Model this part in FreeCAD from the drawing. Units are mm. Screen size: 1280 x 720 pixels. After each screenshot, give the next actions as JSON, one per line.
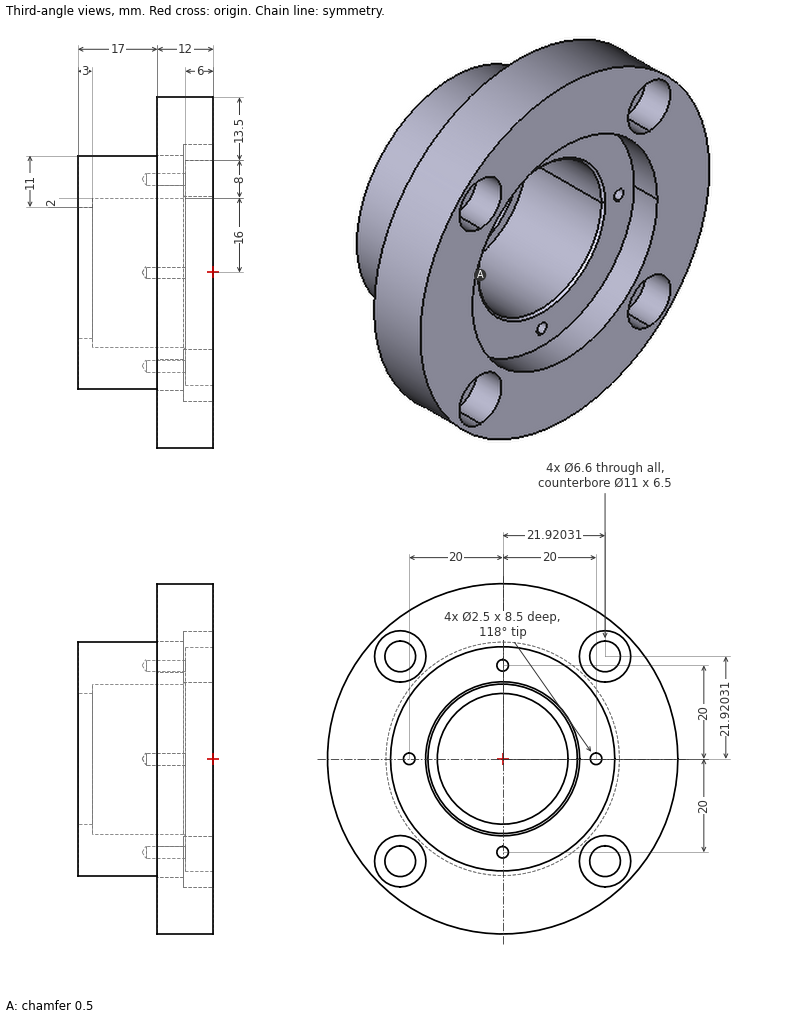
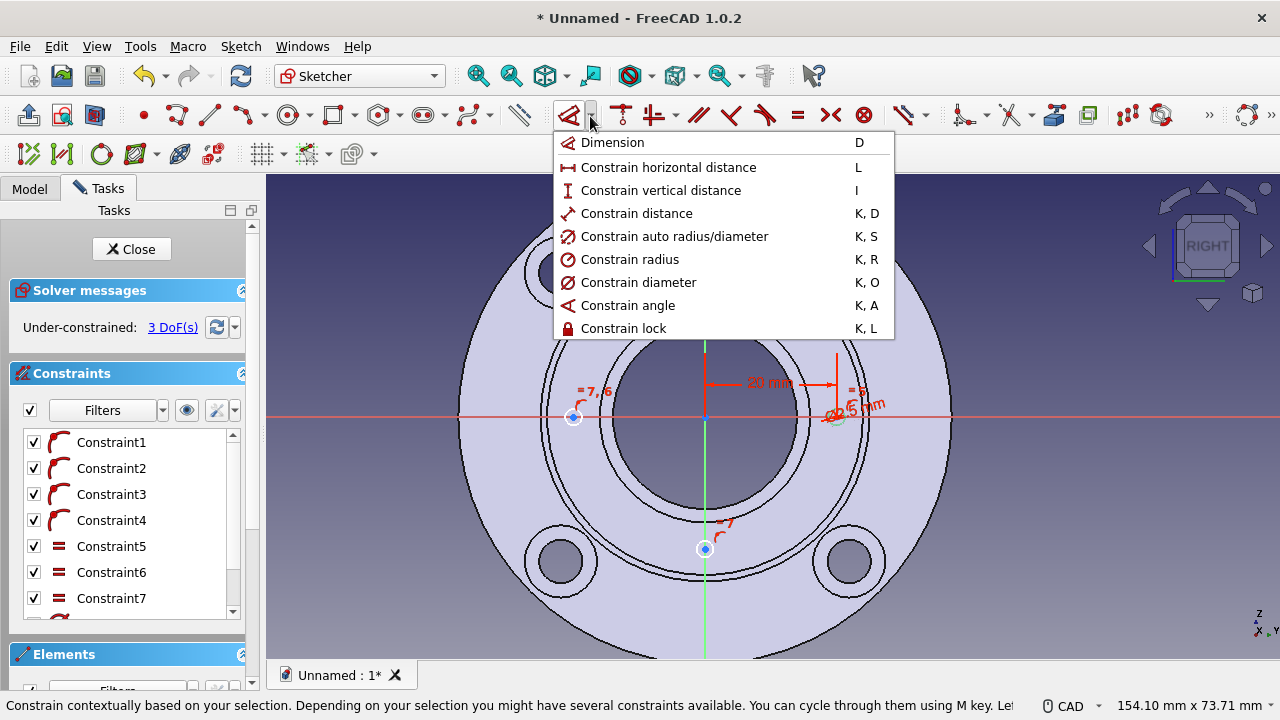
{"action": "left_click", "coordinate": [724, 190]}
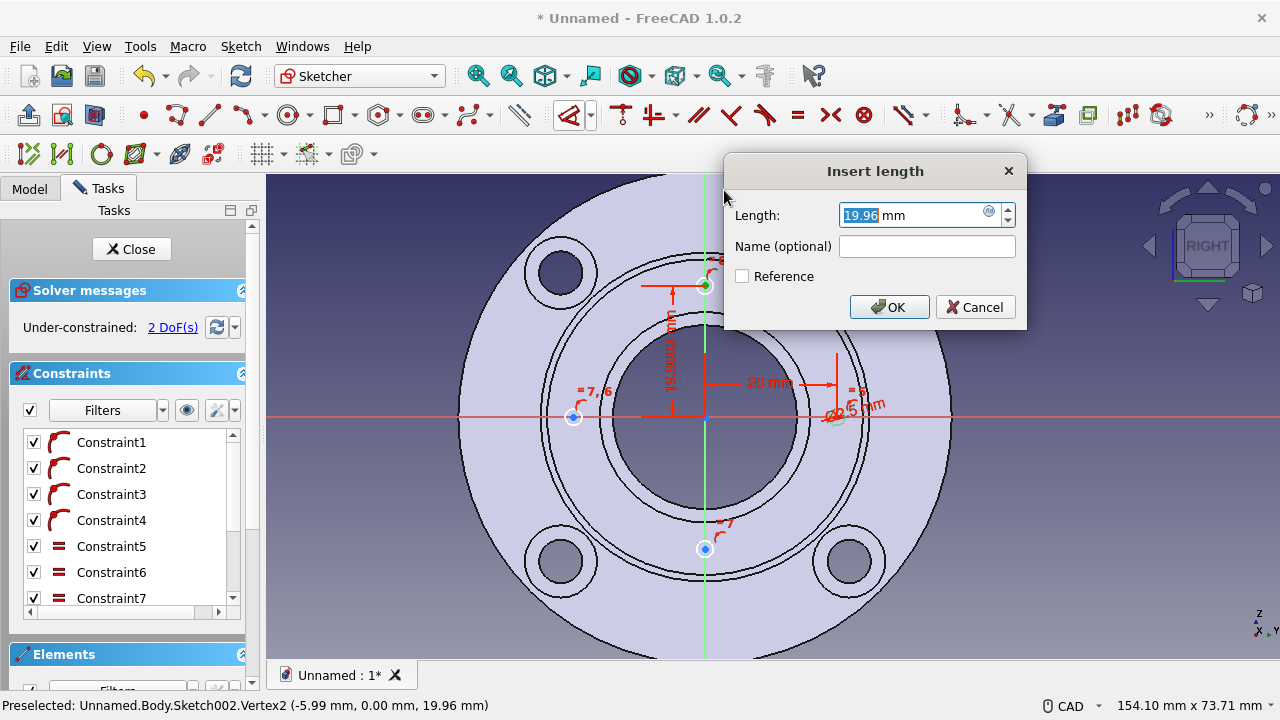
{"action": "type", "text": "20"}
{"action": "key", "text": "Return"}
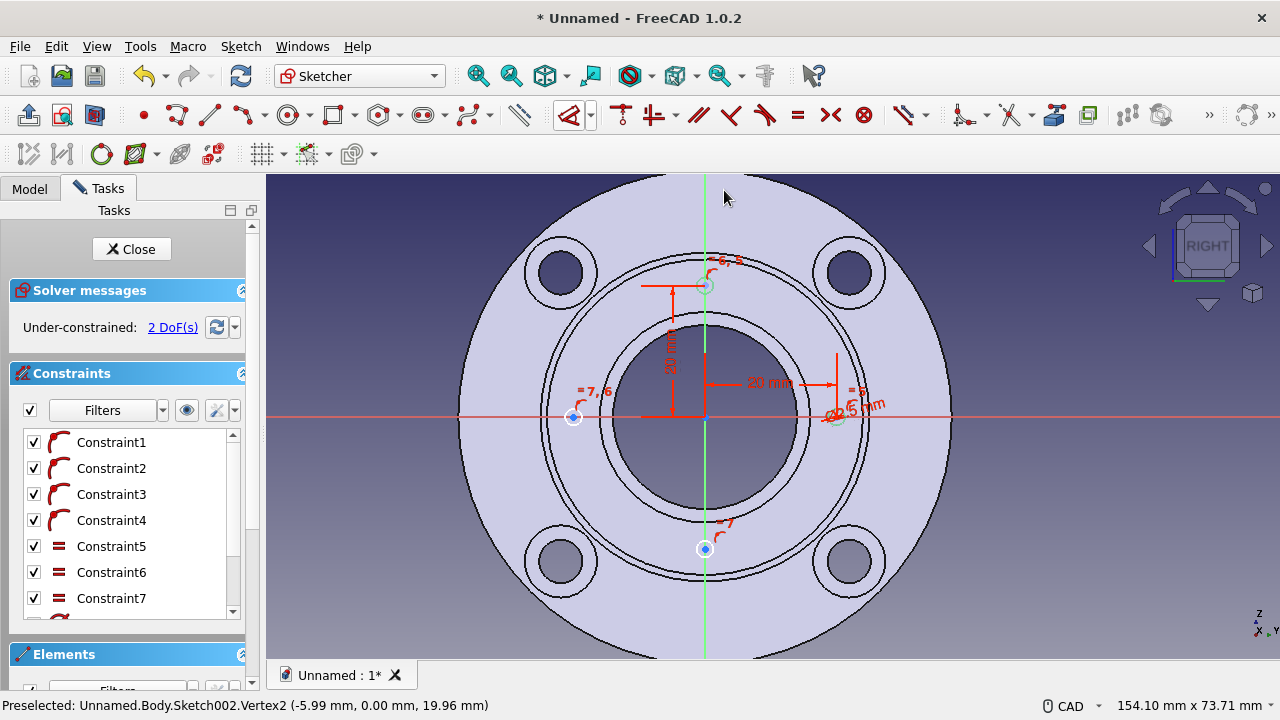
{"action": "left_click", "coordinate": [574, 417]}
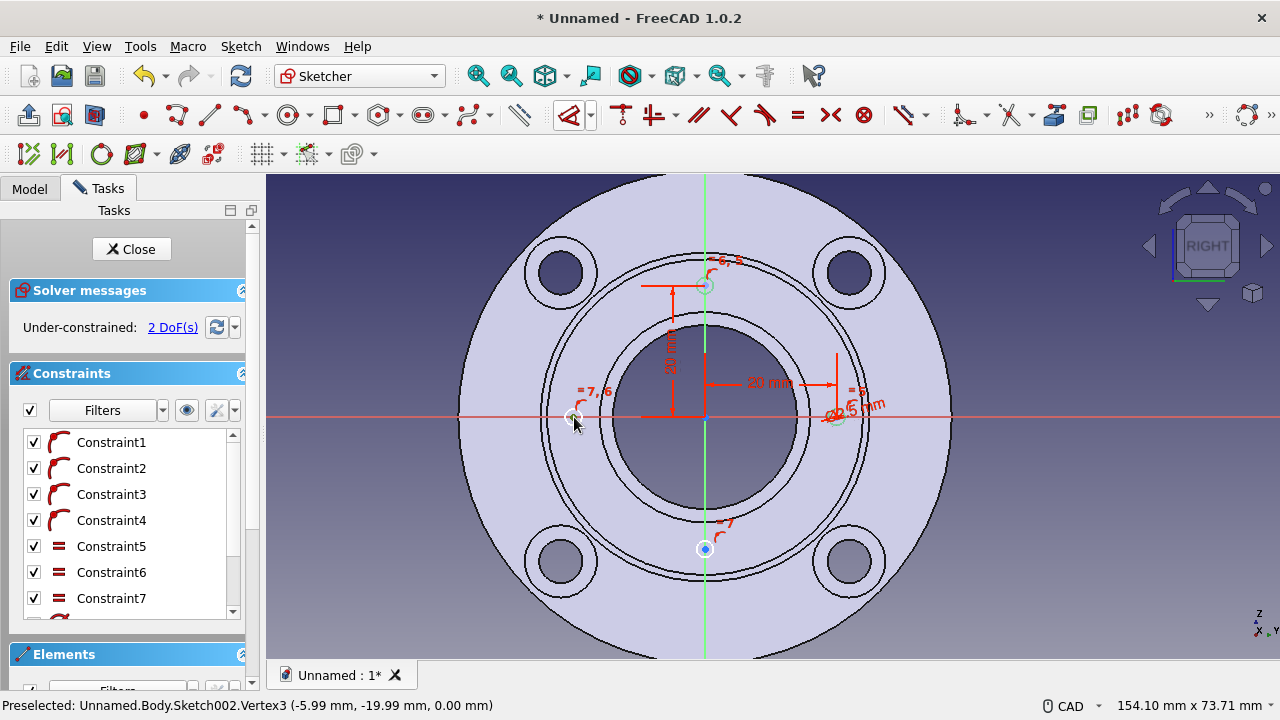
{"action": "left_click", "coordinate": [590, 116]}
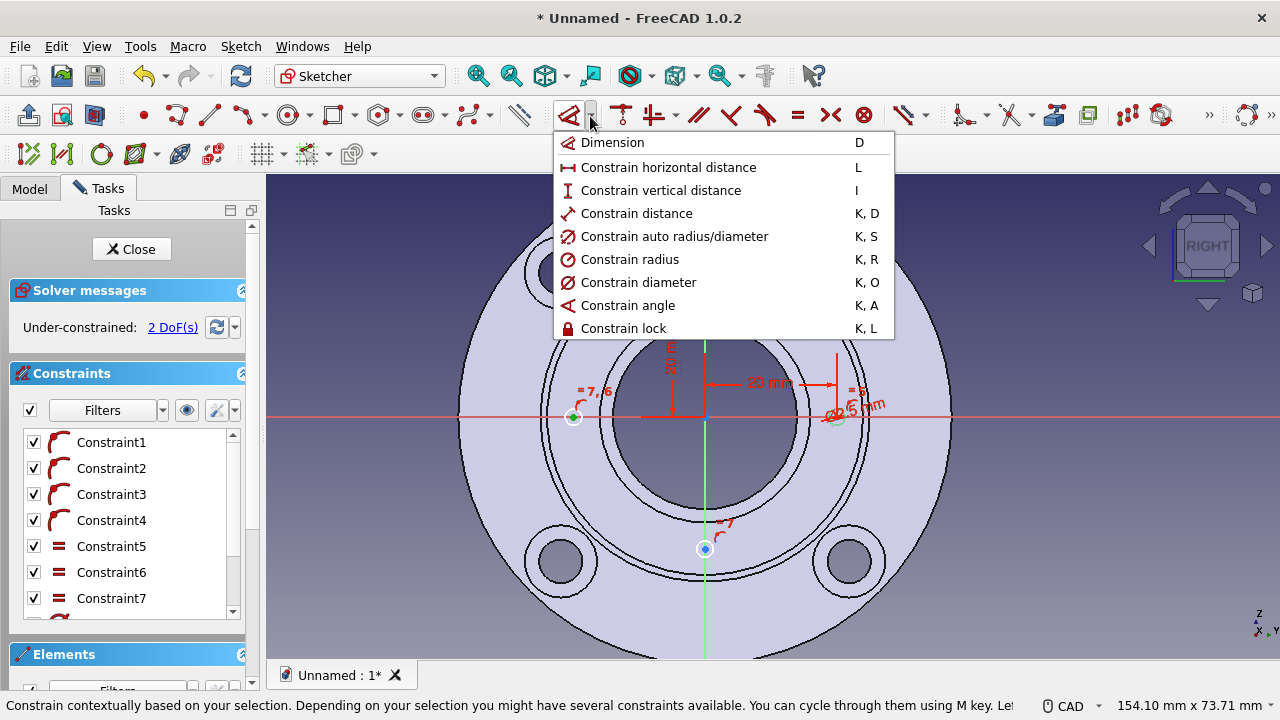
{"action": "left_click", "coordinate": [724, 168]}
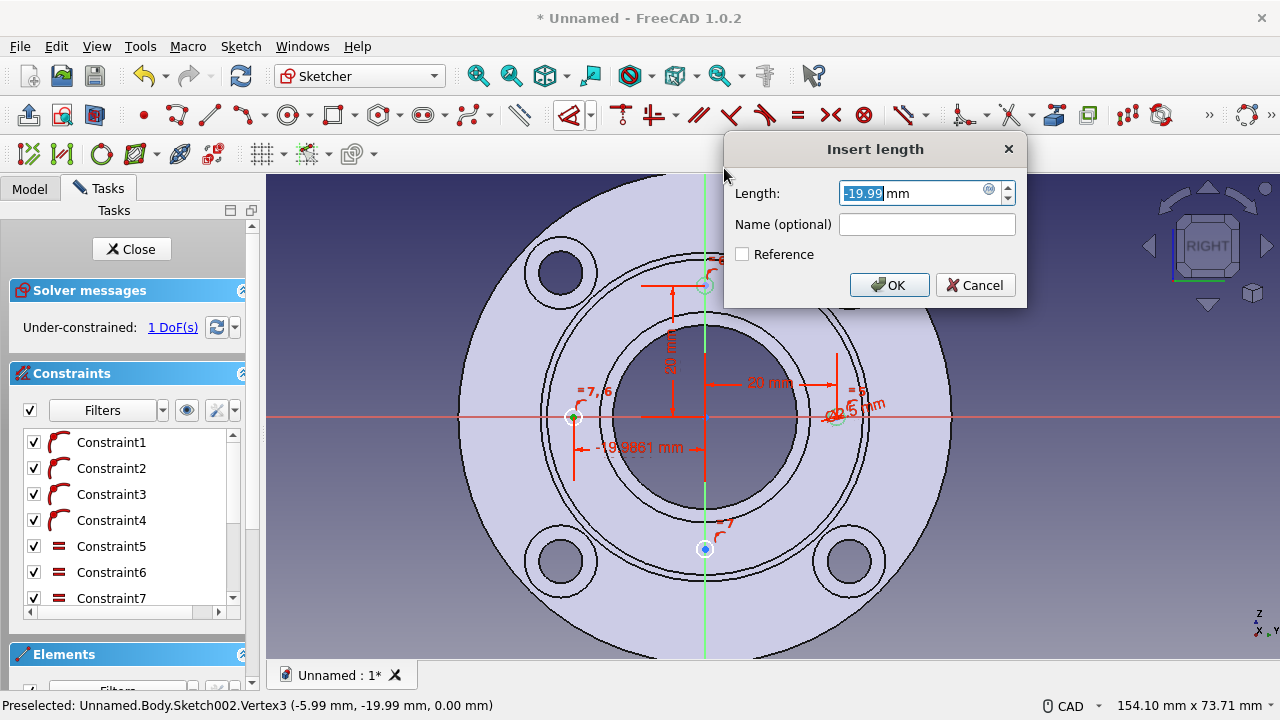
{"action": "type", "text": "-20"}
{"action": "key", "text": "Return"}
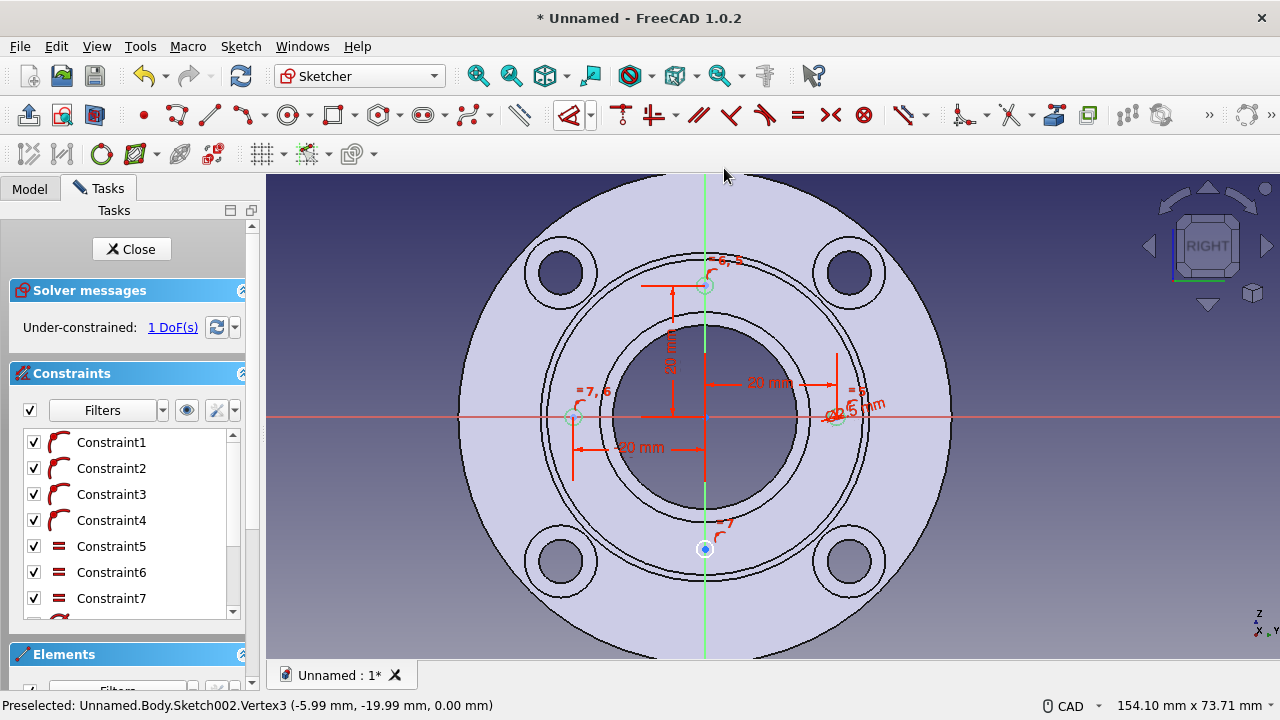
{"action": "left_click", "coordinate": [705, 549]}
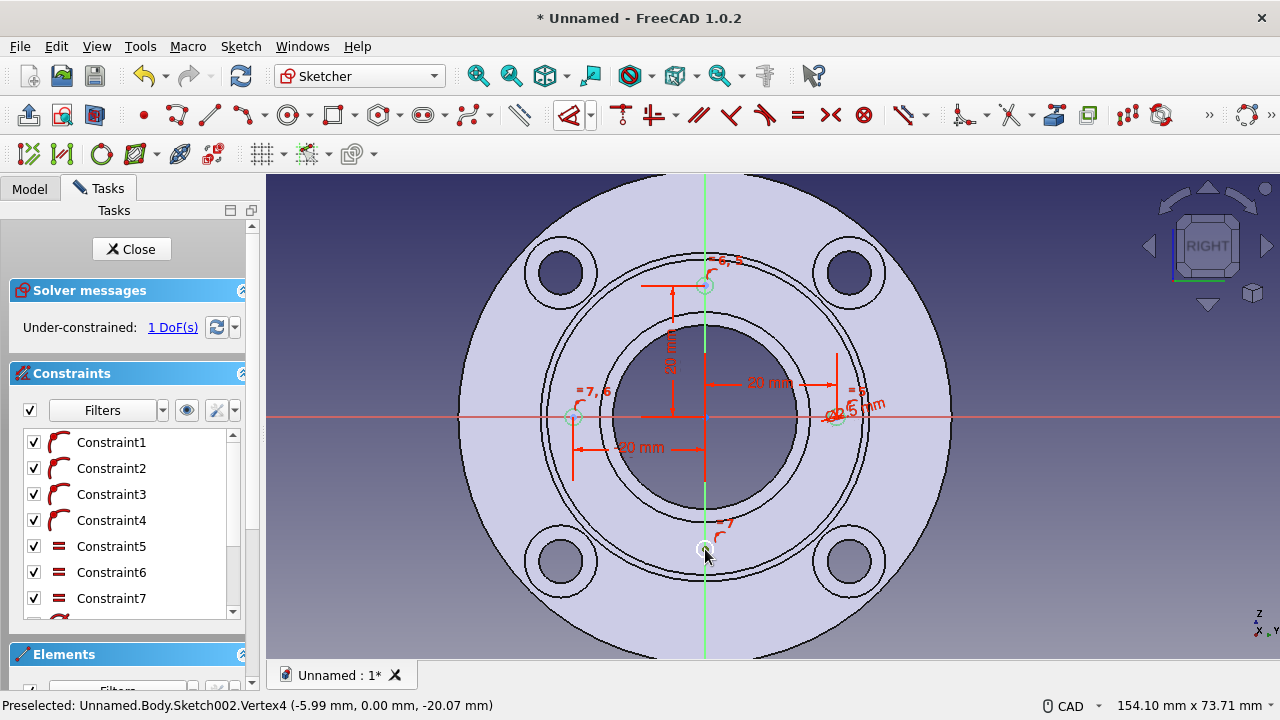
{"action": "key", "text": "i"}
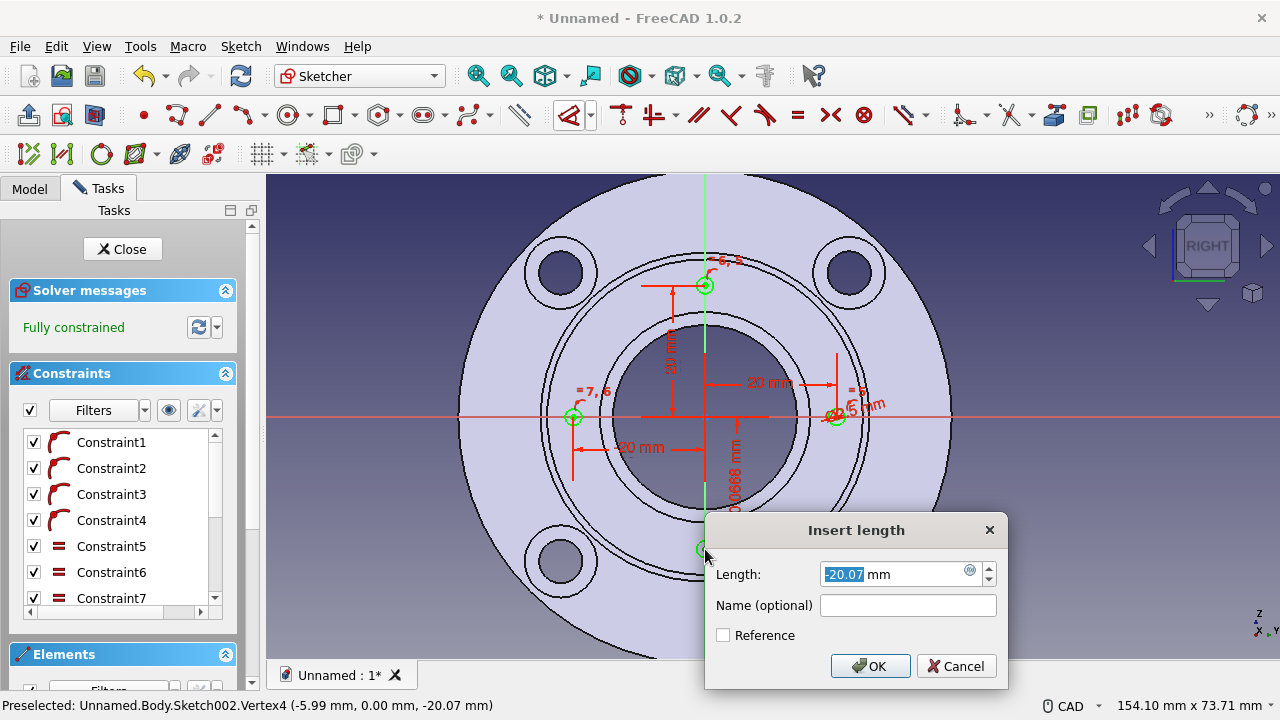
{"action": "type", "text": "-20"}
{"action": "key", "text": "Return"}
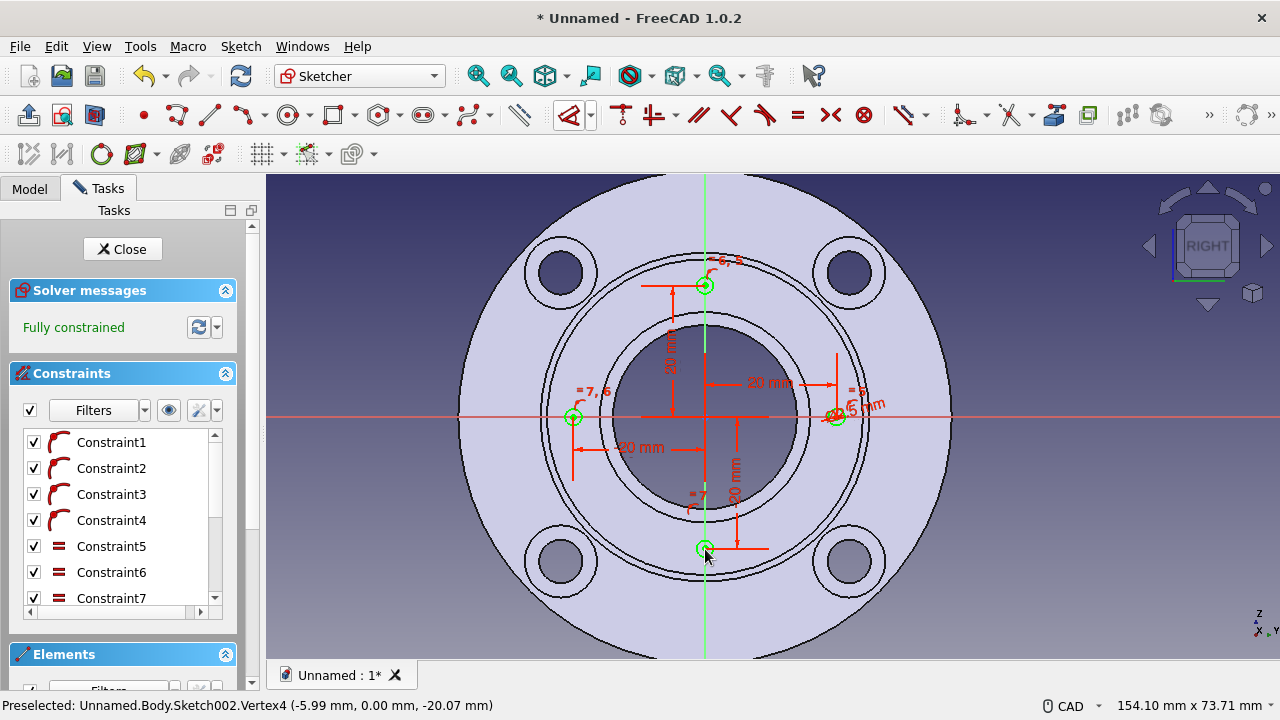
{"action": "left_click", "coordinate": [123, 249]}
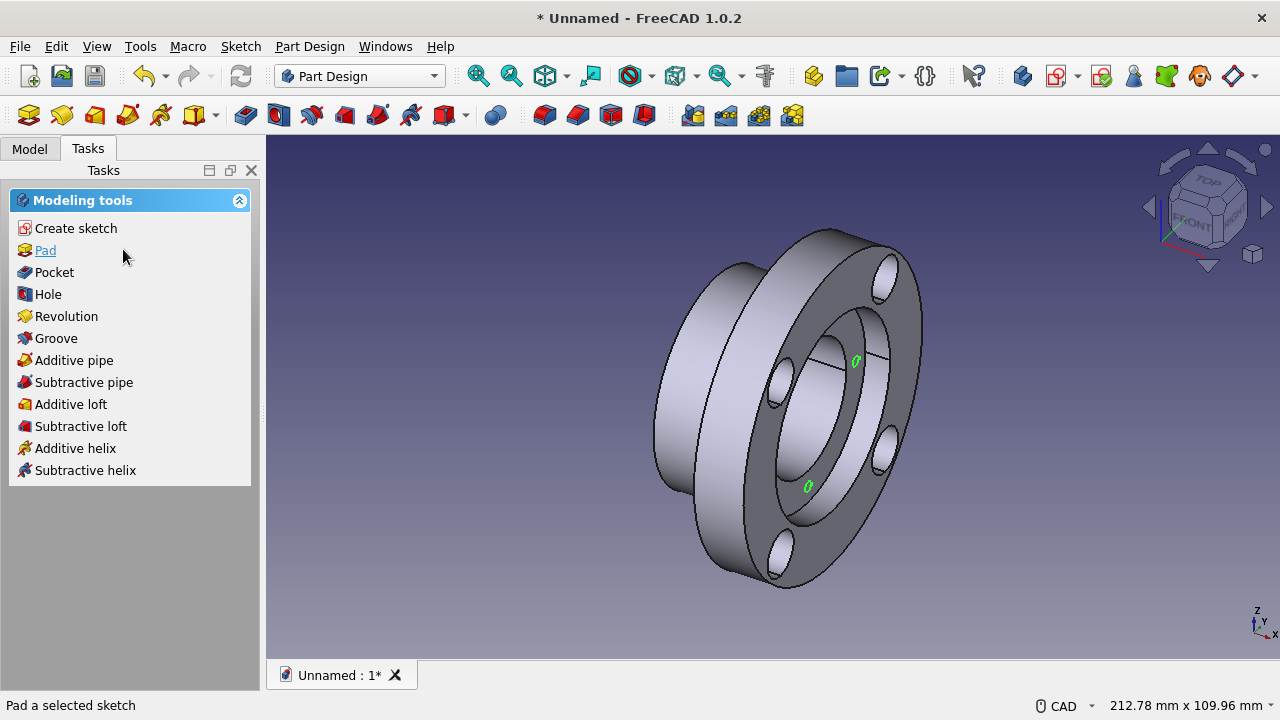
{"action": "left_click", "coordinate": [279, 116]}